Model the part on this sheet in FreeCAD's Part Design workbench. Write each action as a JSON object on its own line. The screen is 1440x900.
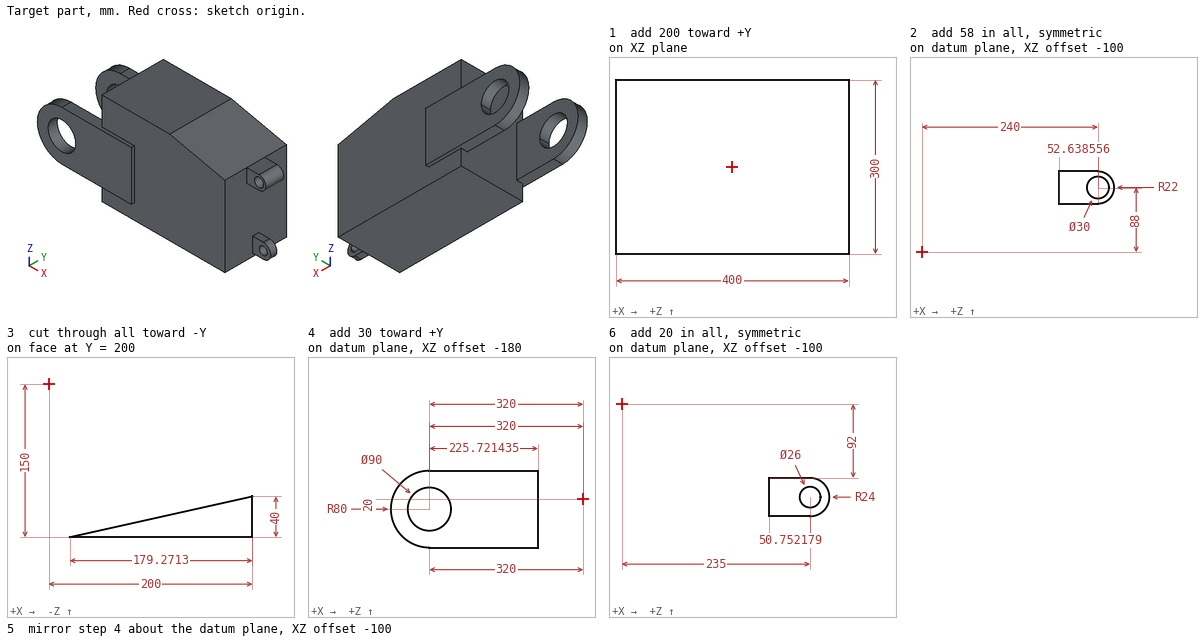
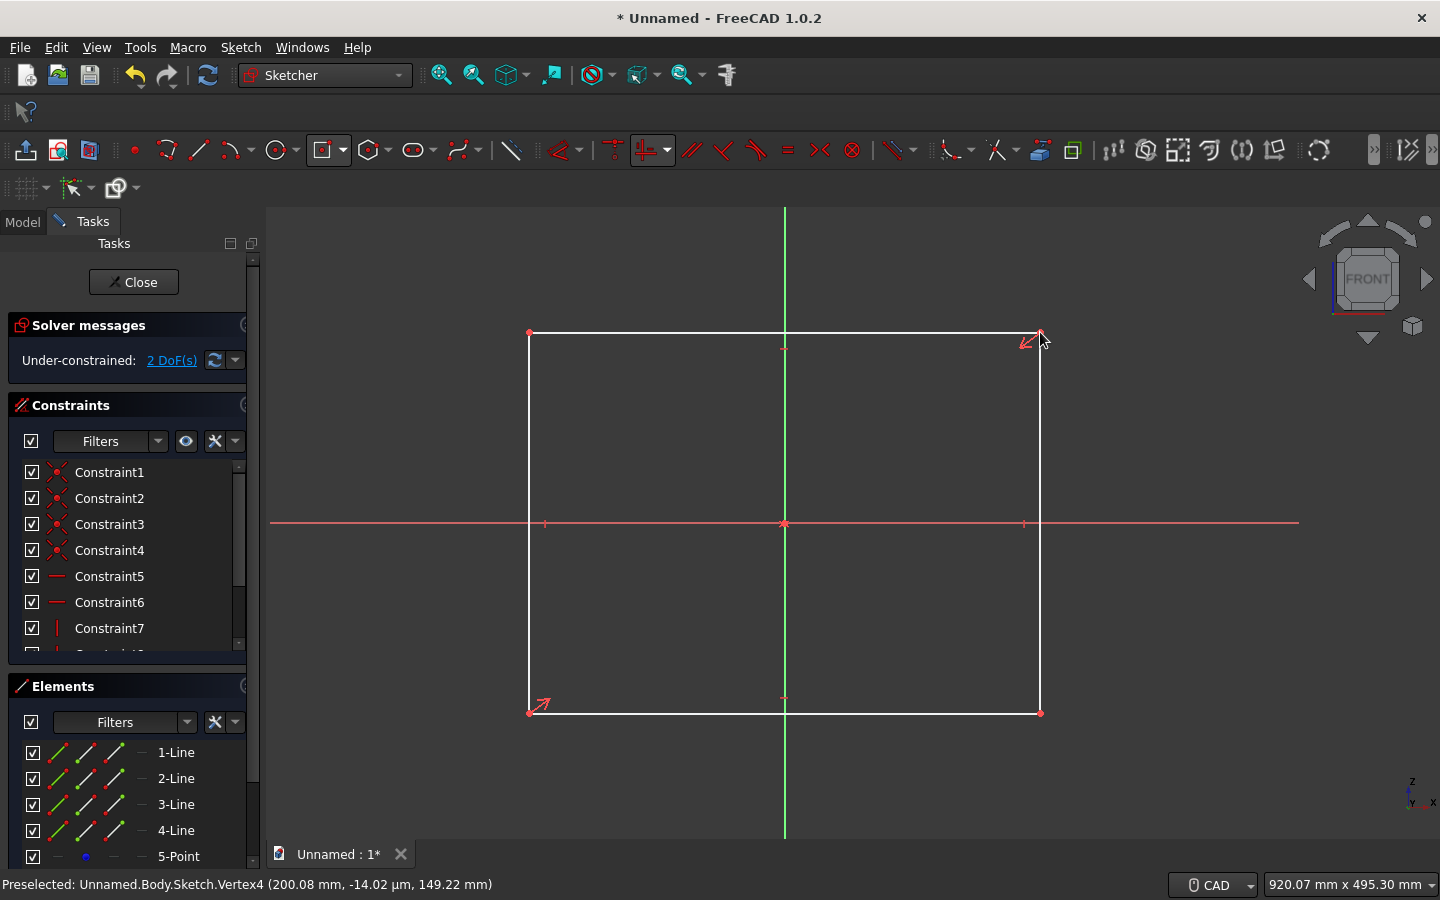
{"action": "left_click", "coordinate": [683, 714]}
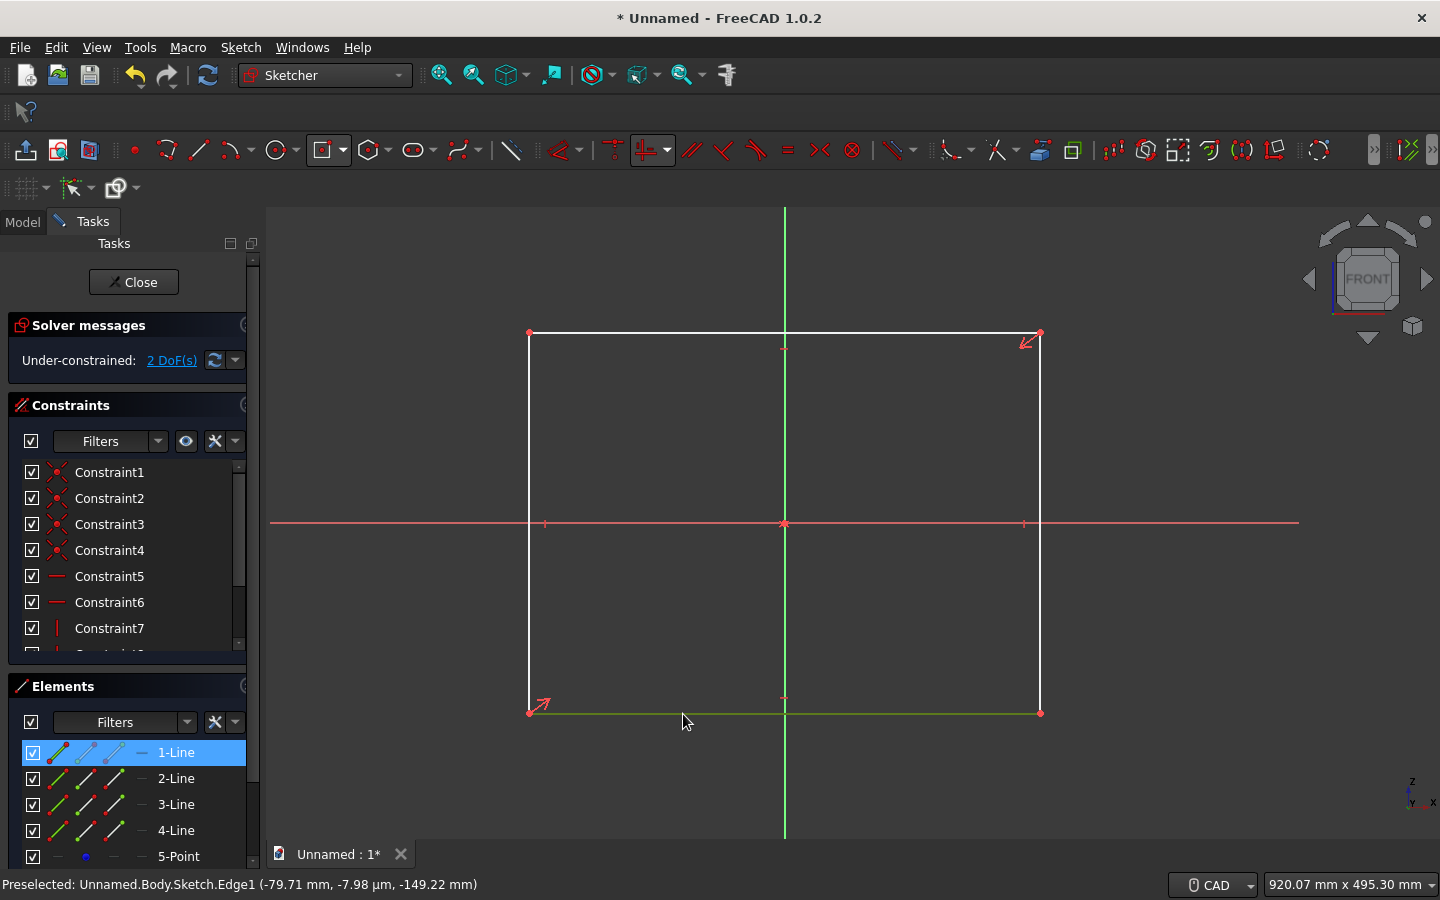
{"action": "left_click", "coordinate": [582, 150]}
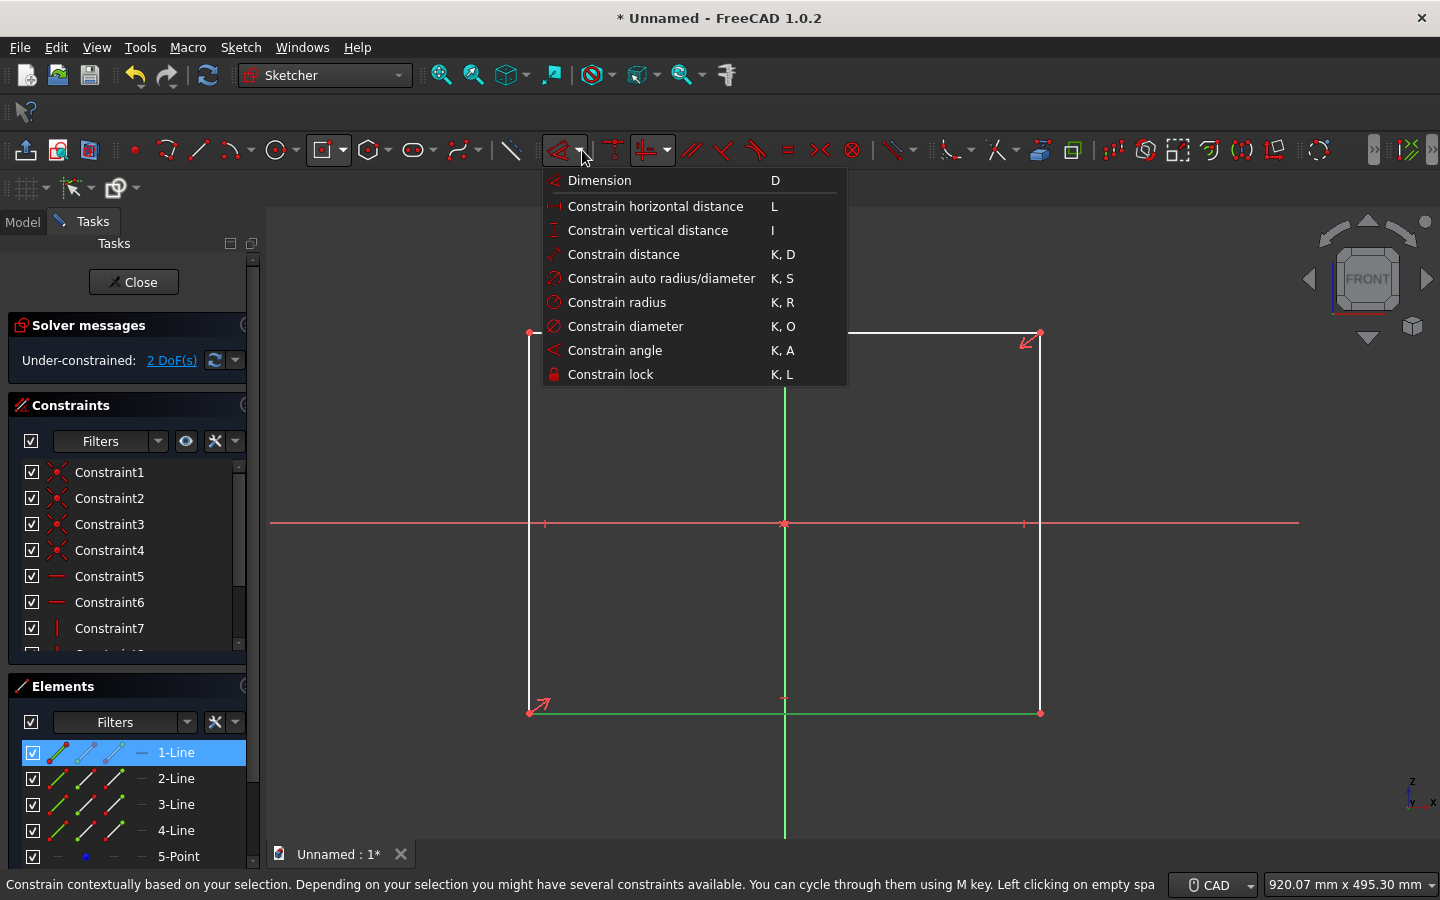
{"action": "left_click", "coordinate": [695, 206]}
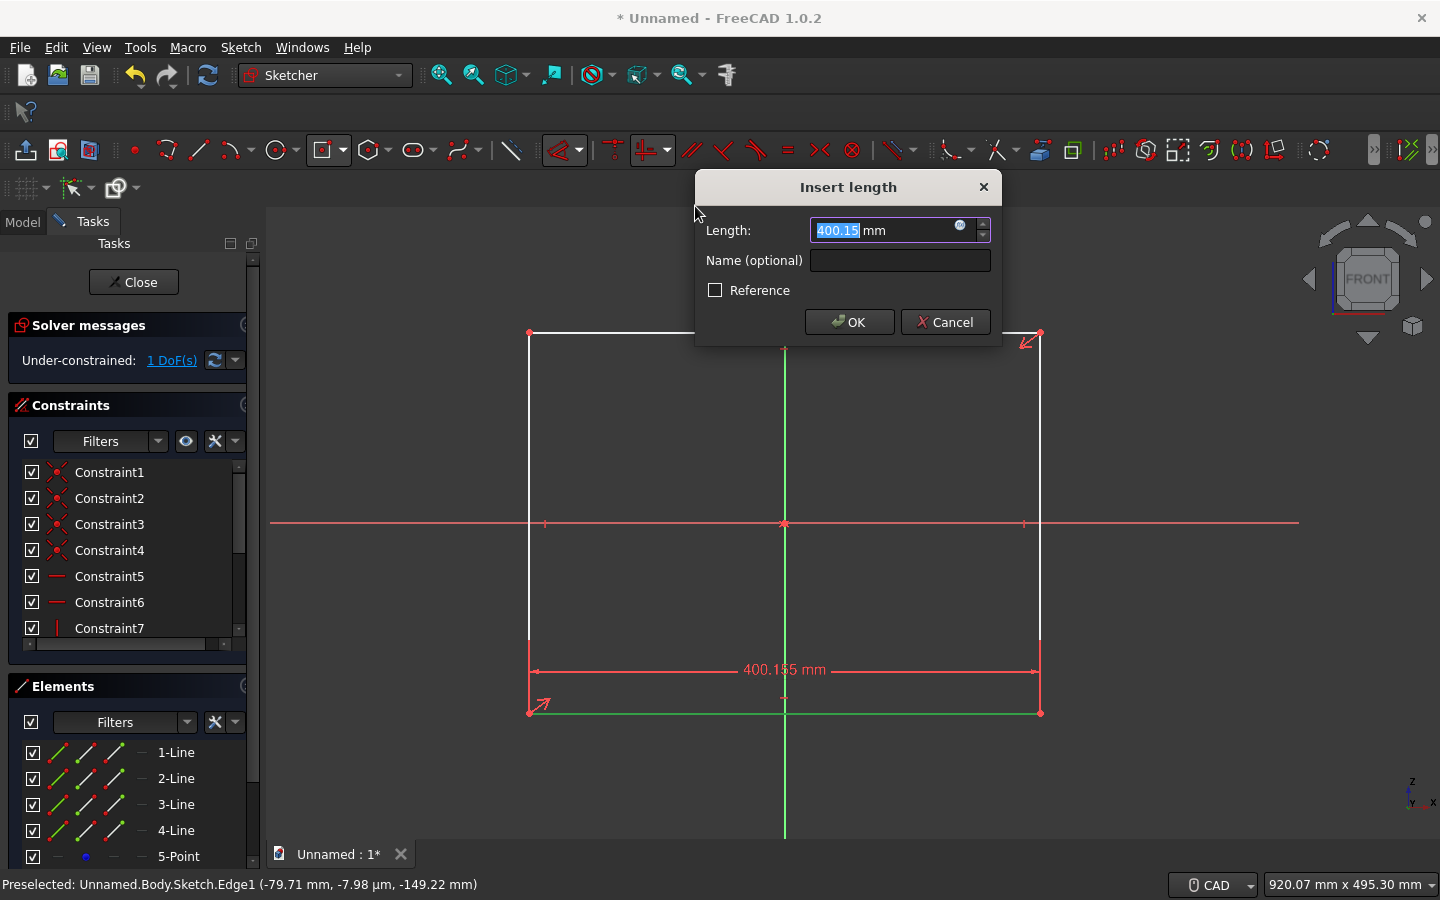
{"action": "type", "text": "400"}
{"action": "key", "text": "Return"}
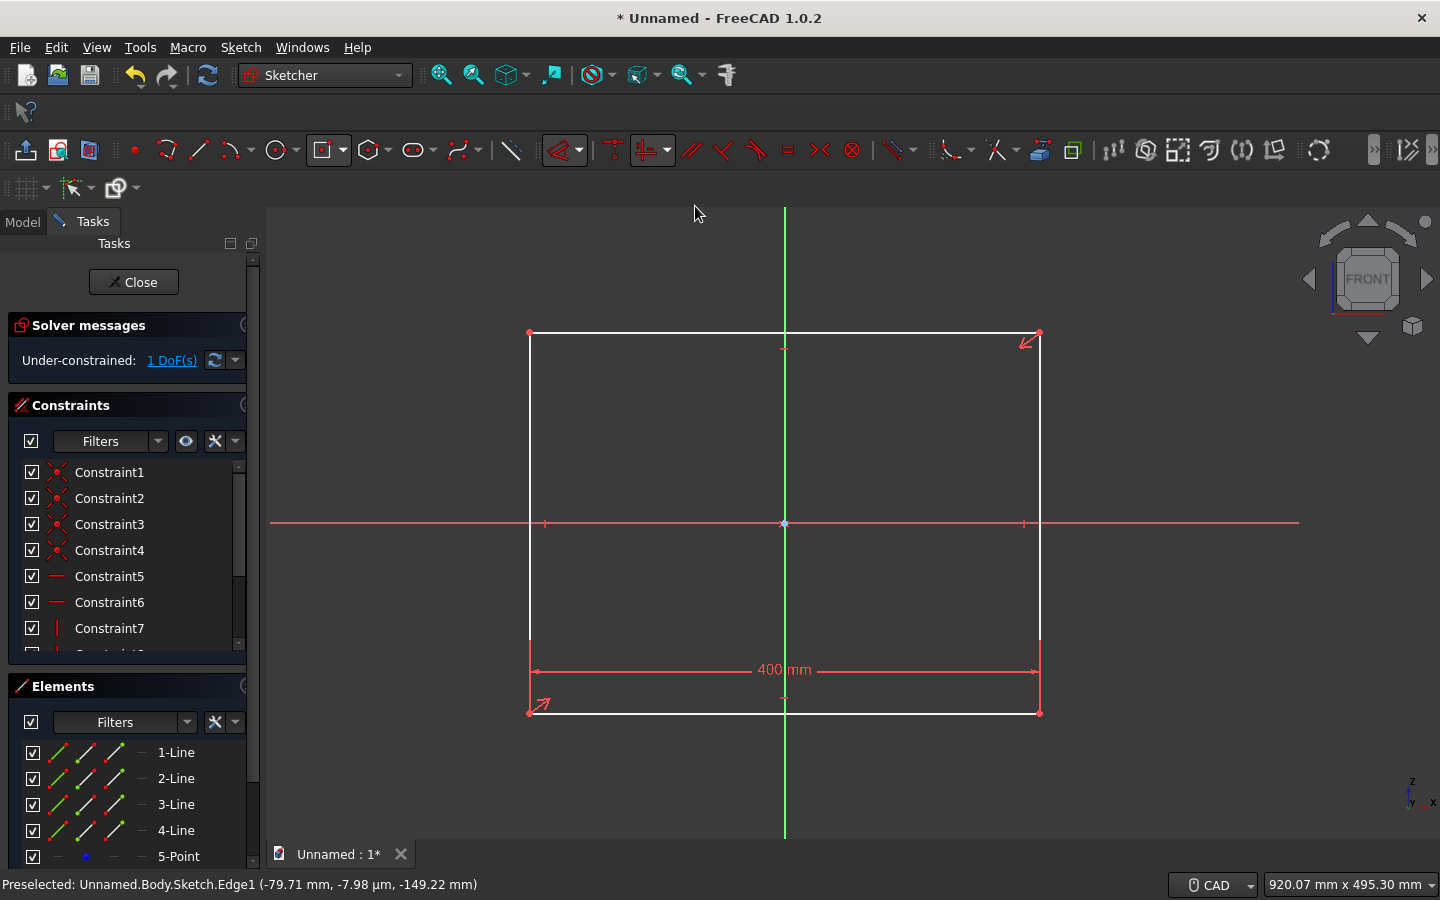
{"action": "left_click", "coordinate": [1040, 600]}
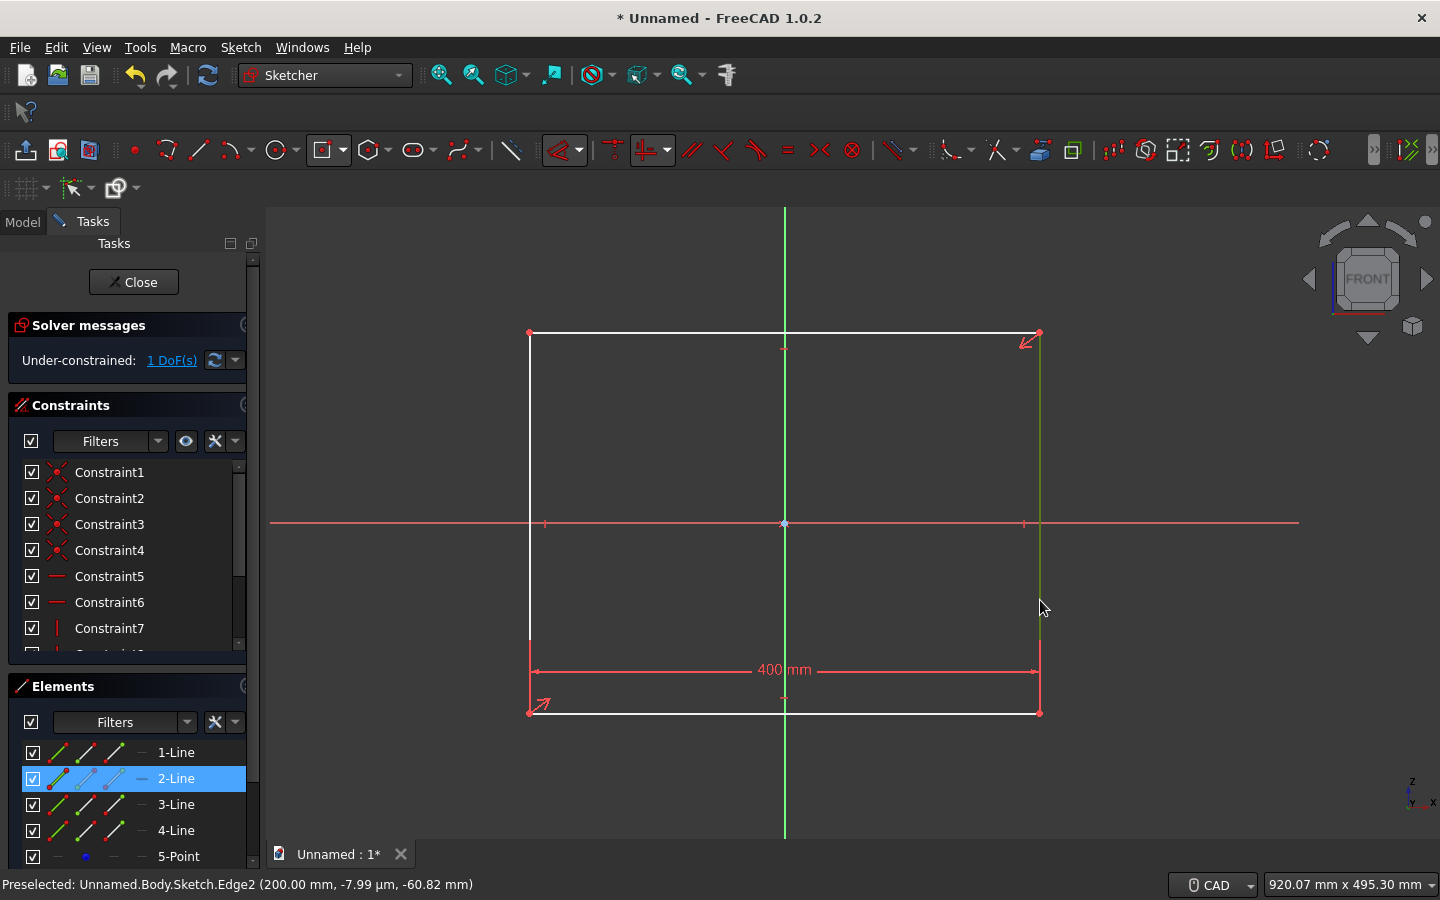
{"action": "left_click", "coordinate": [582, 150]}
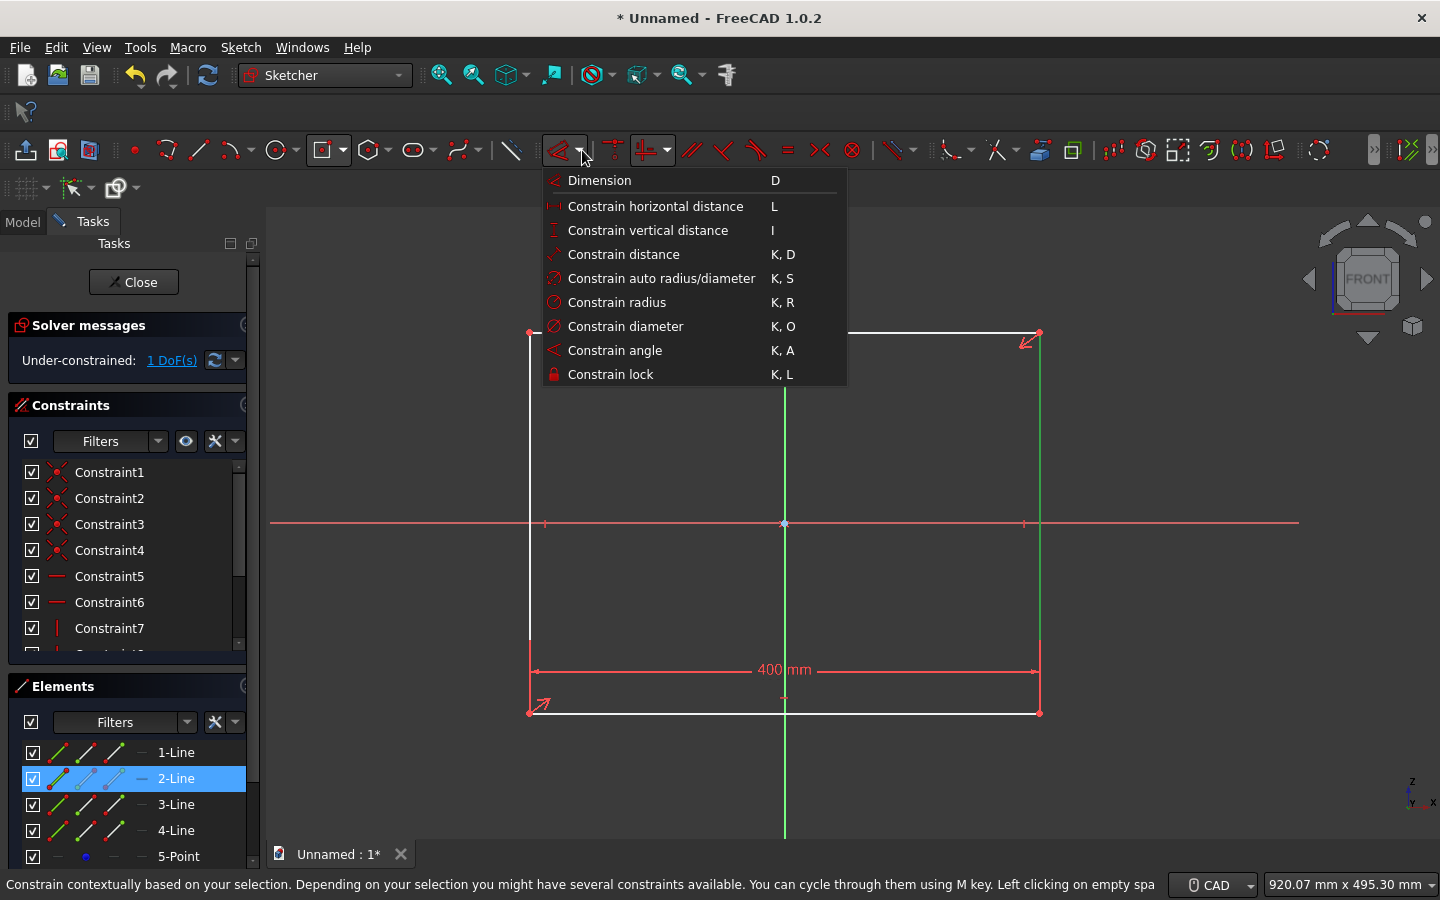
{"action": "left_click", "coordinate": [695, 230]}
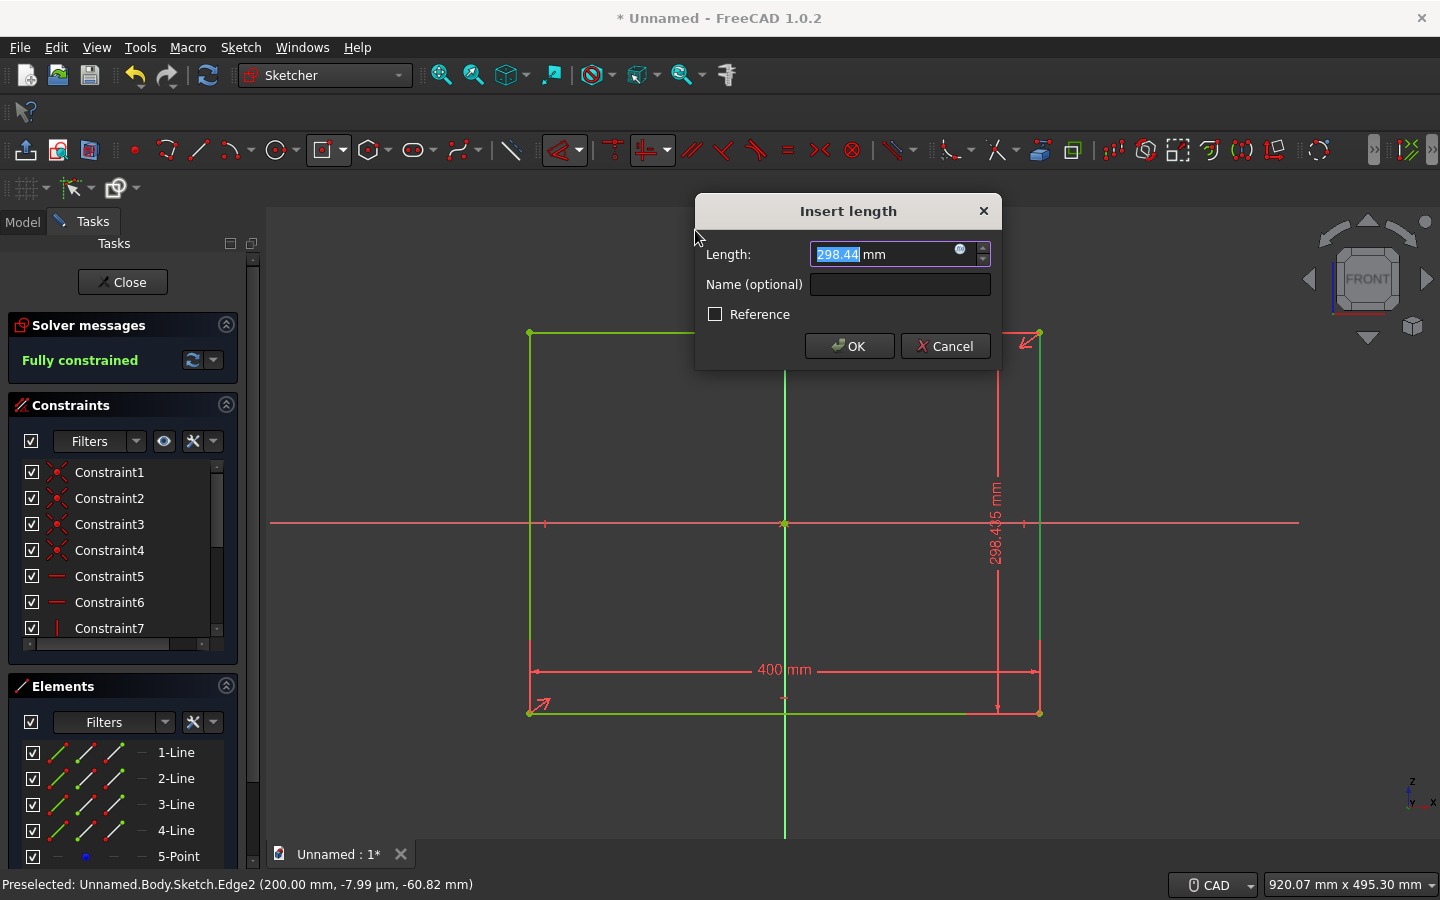
{"action": "type", "text": "300"}
{"action": "key", "text": "Return"}